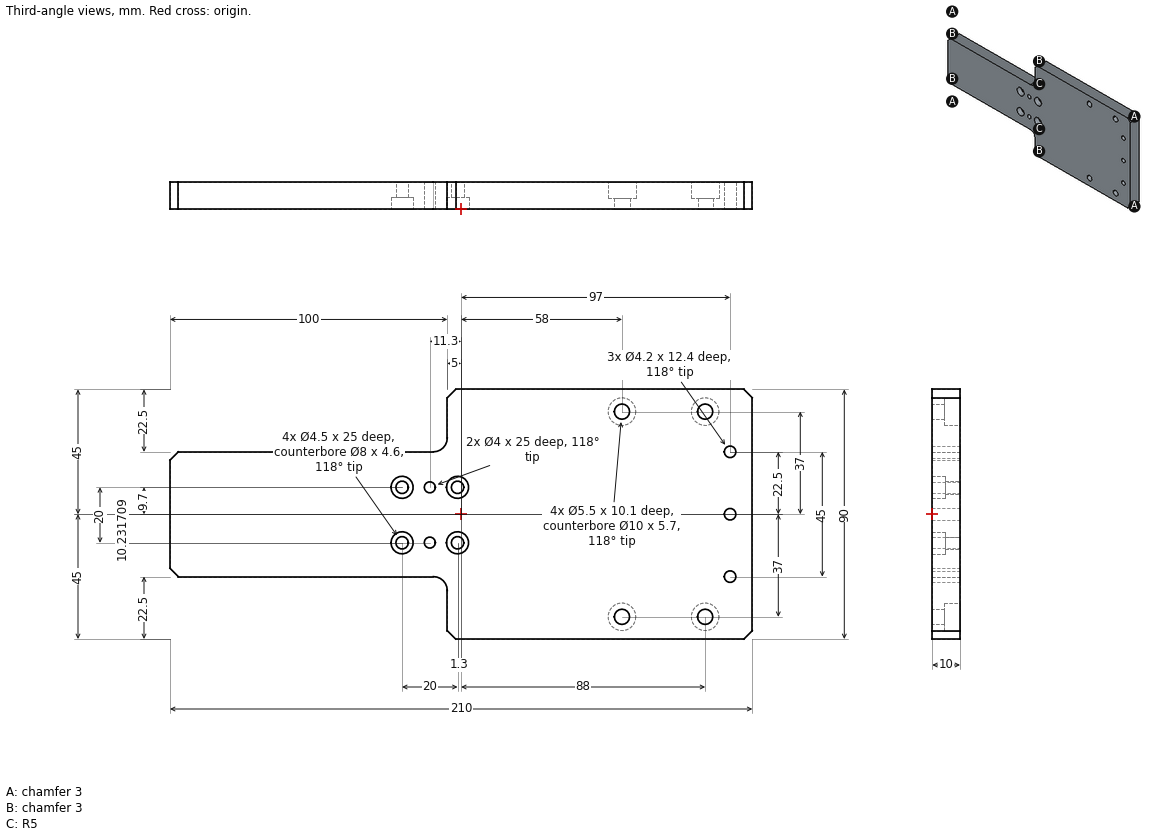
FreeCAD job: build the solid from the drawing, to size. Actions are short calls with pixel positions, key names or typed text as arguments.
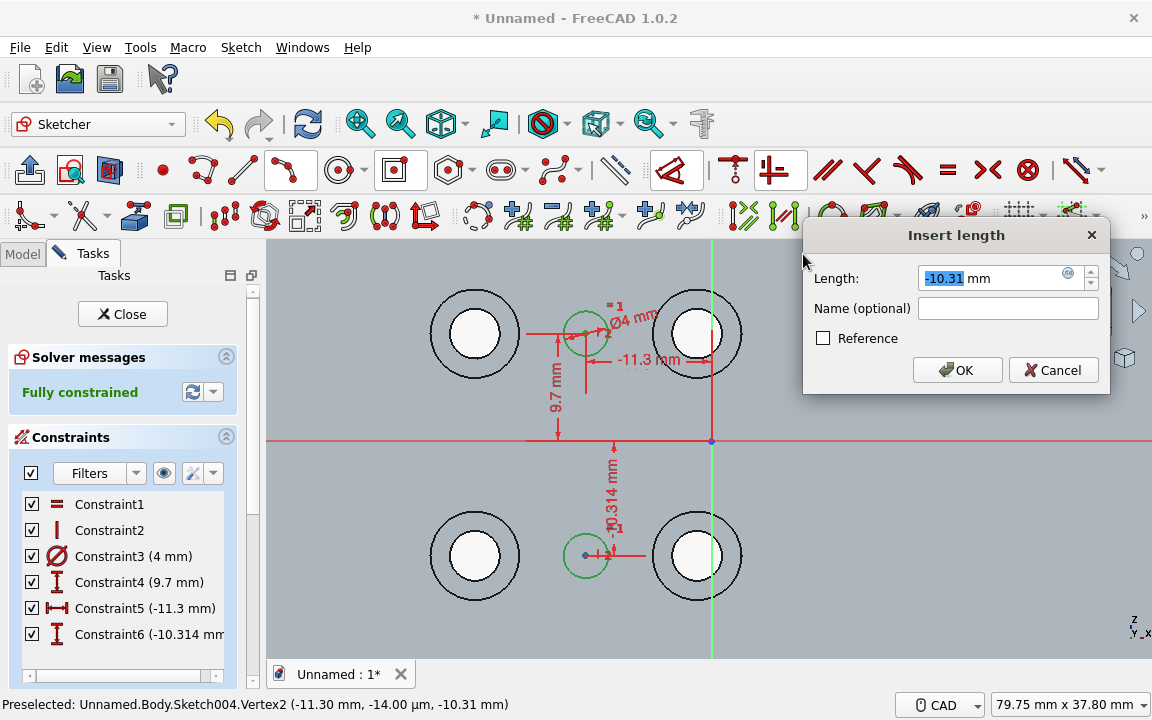
text(-10.231709)
key(Return)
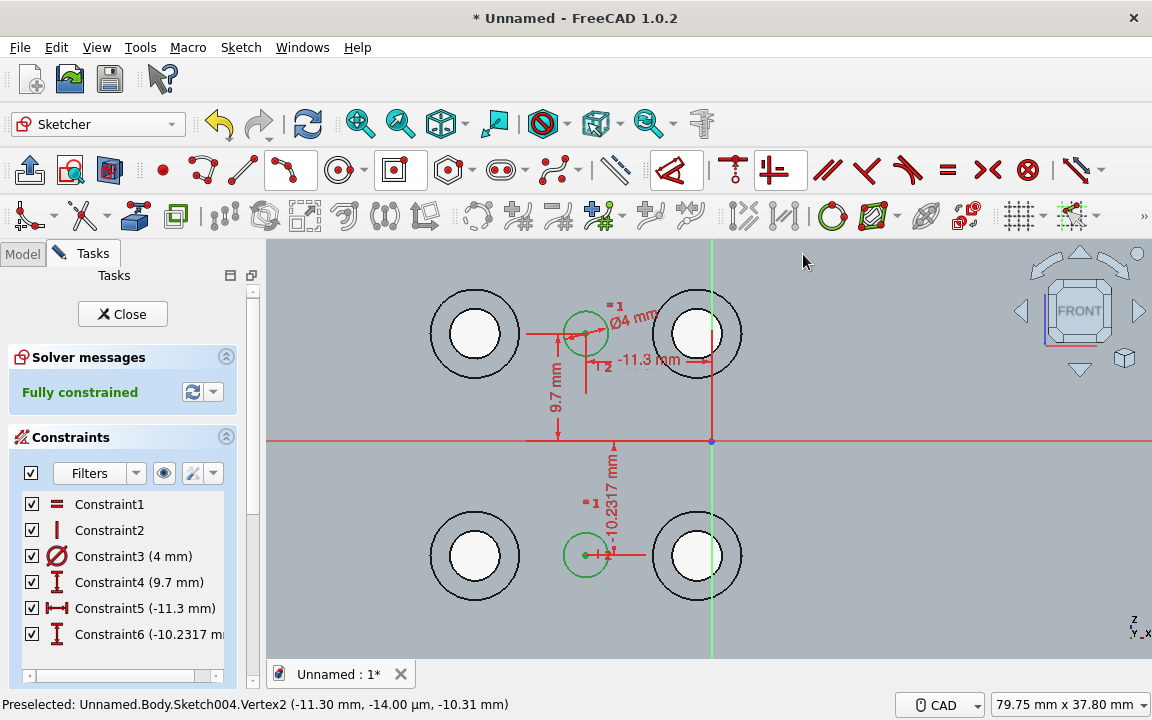
click(123, 314)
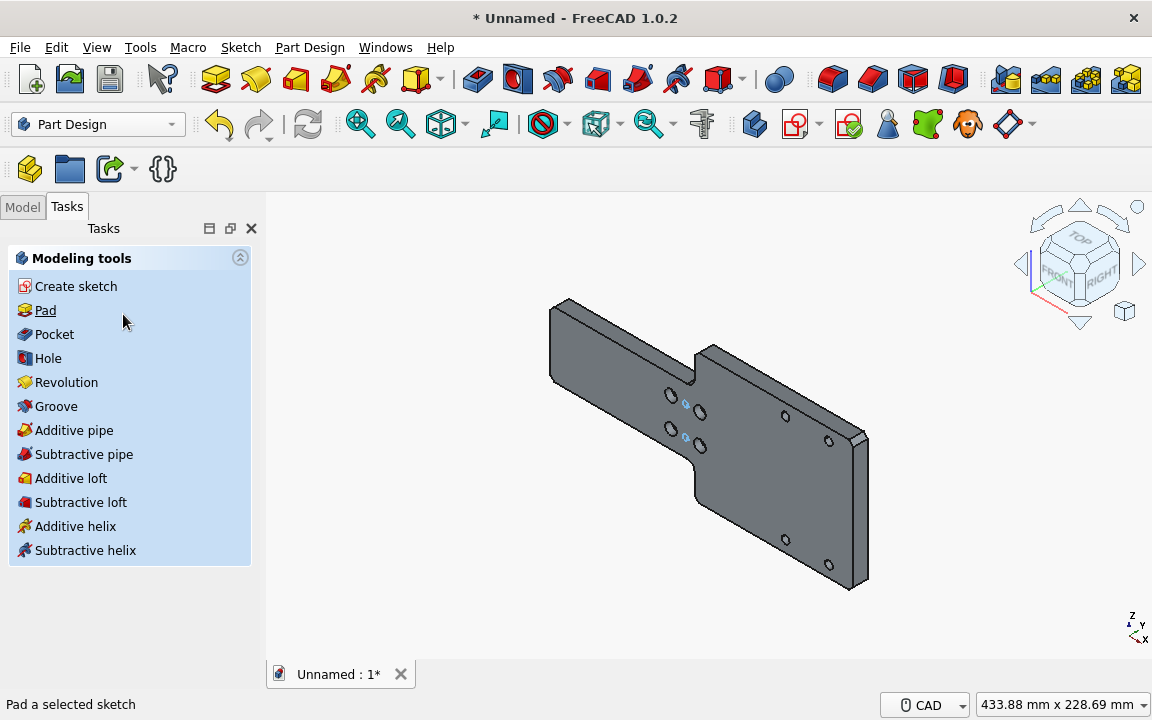
click(518, 80)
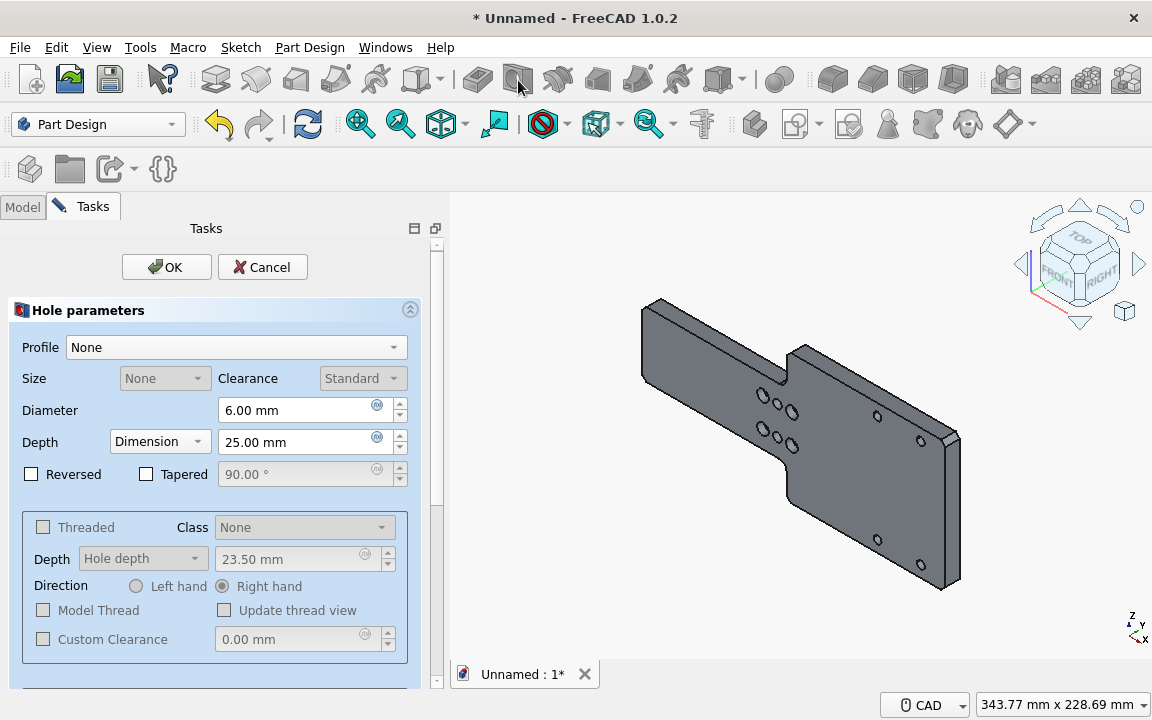
triple_click(305, 410)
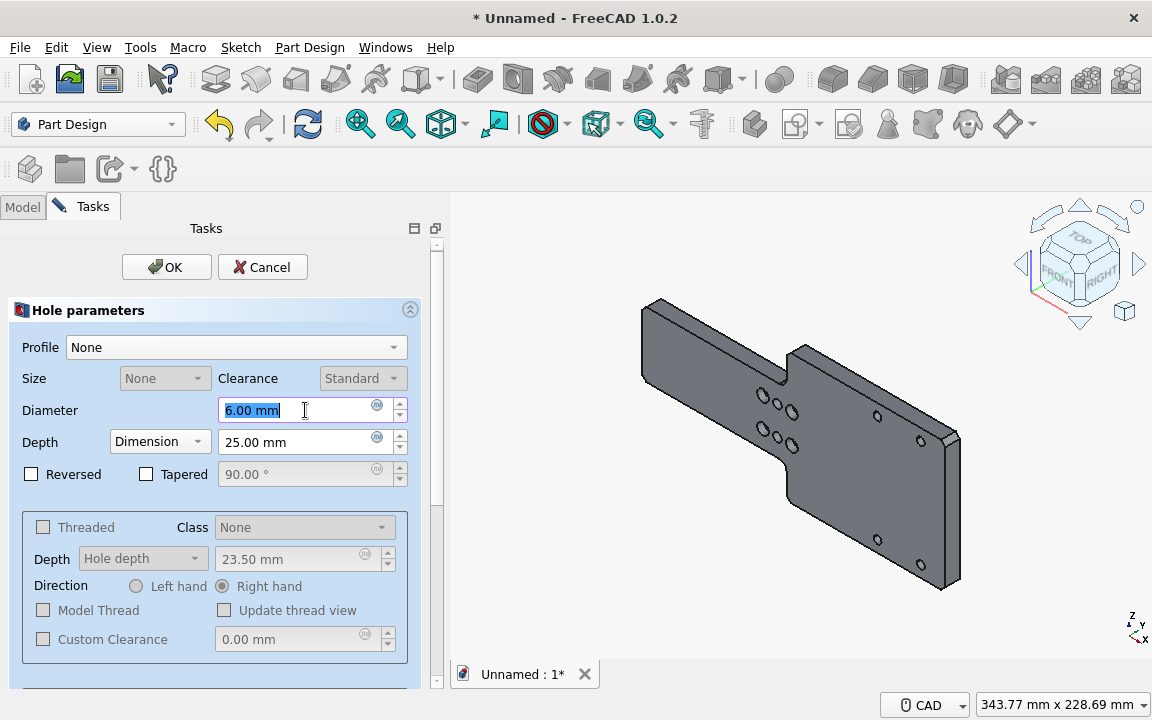
text(4)
key(Tab)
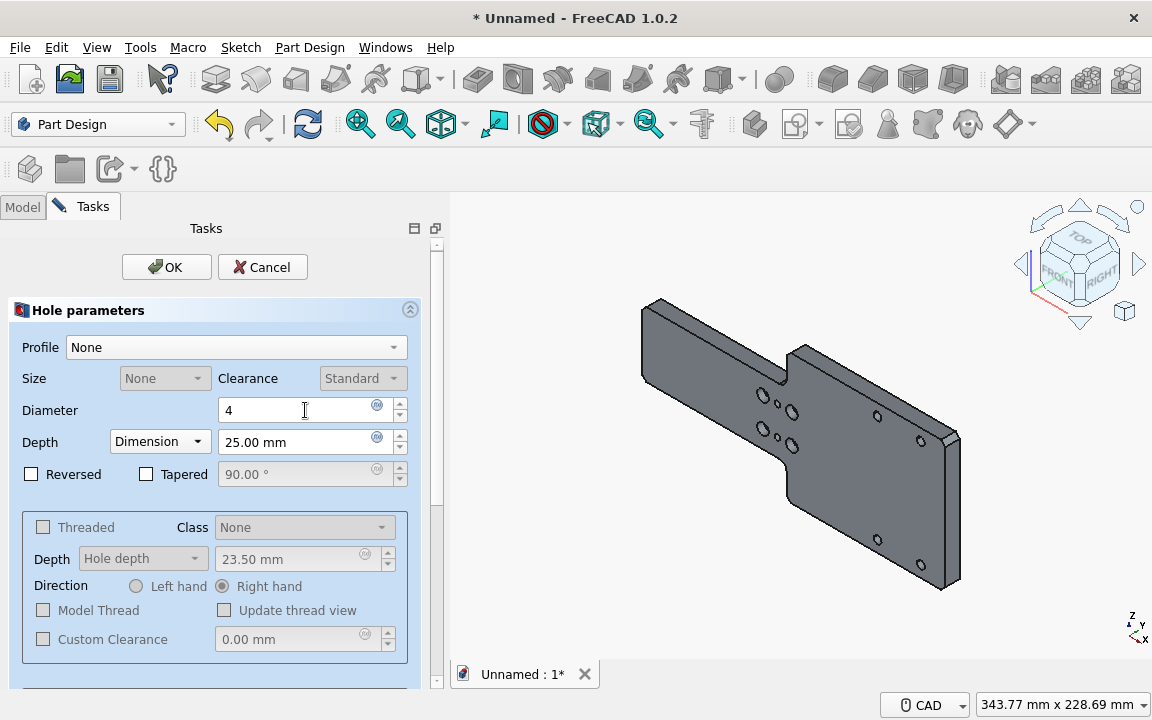
triple_click(305, 442)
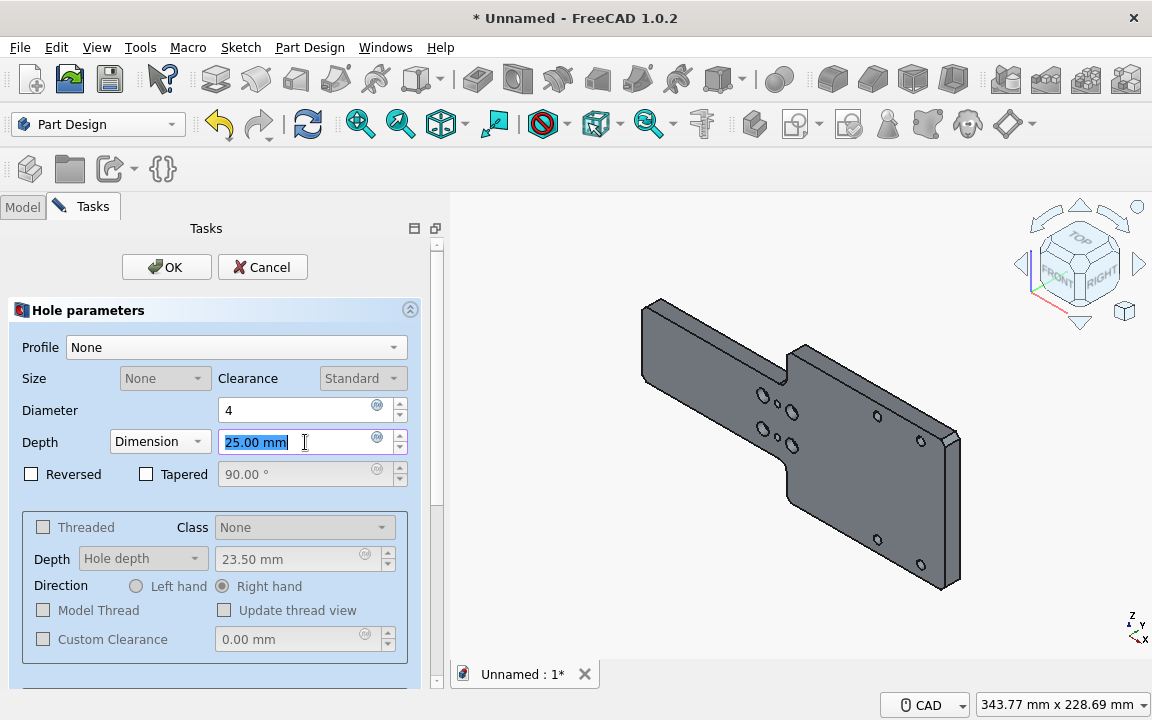
text(25)
key(Tab)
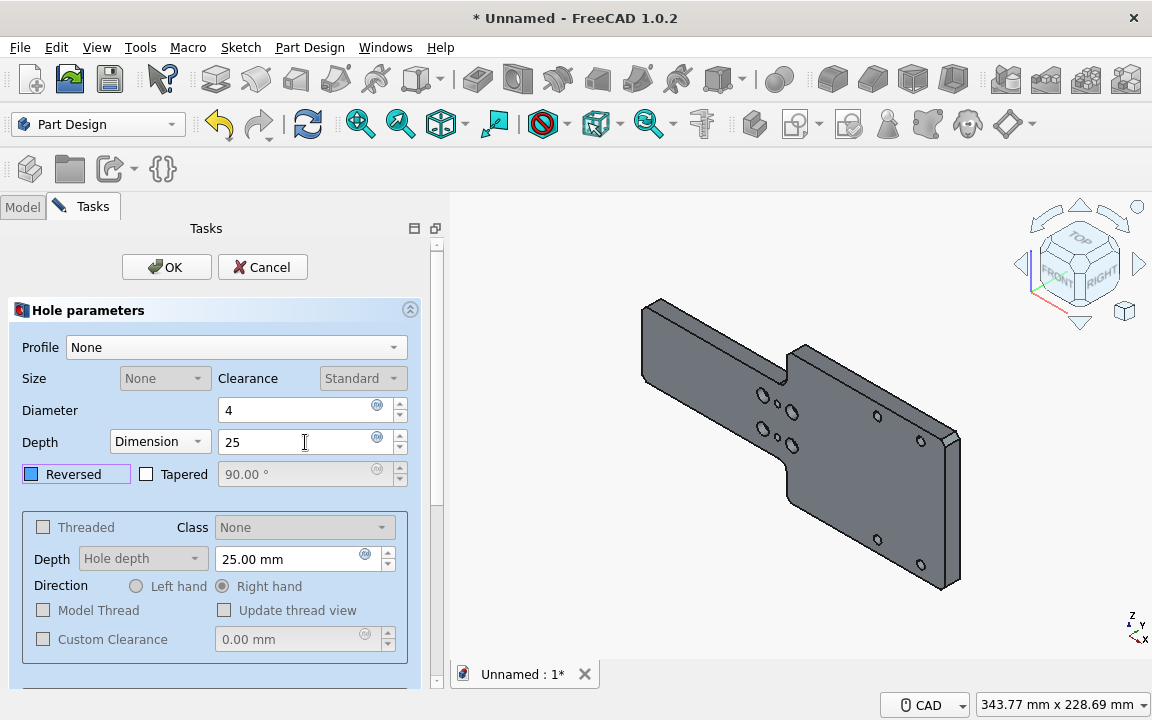
click(167, 267)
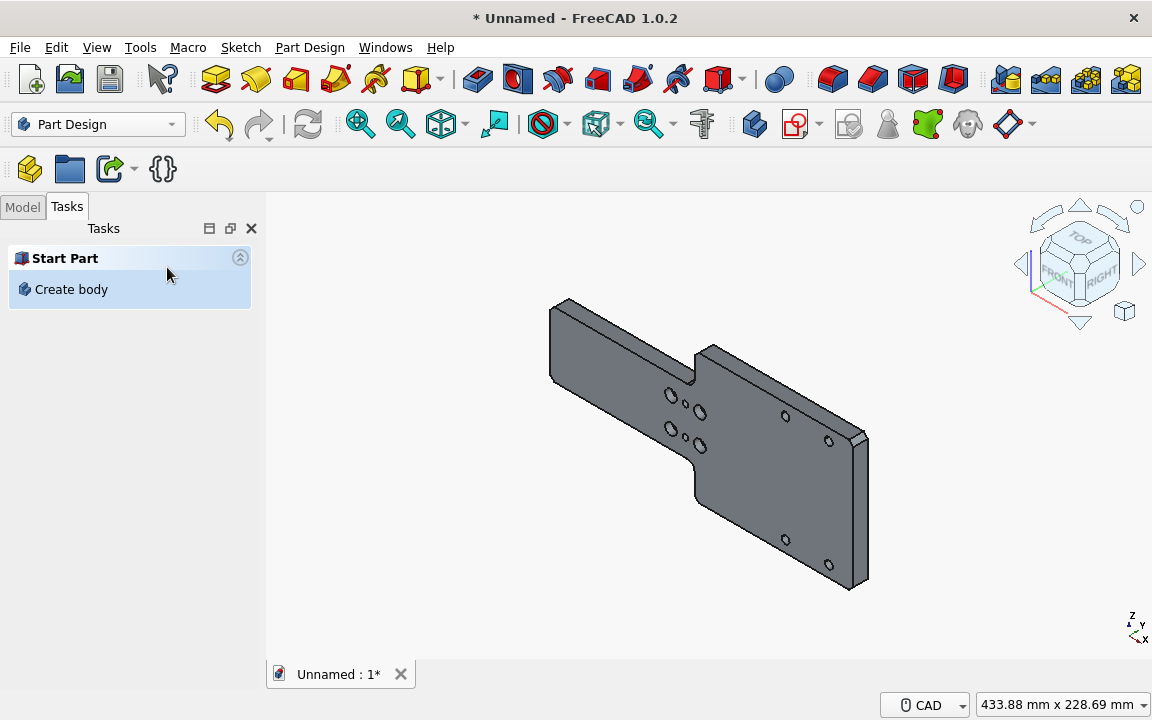
key(4)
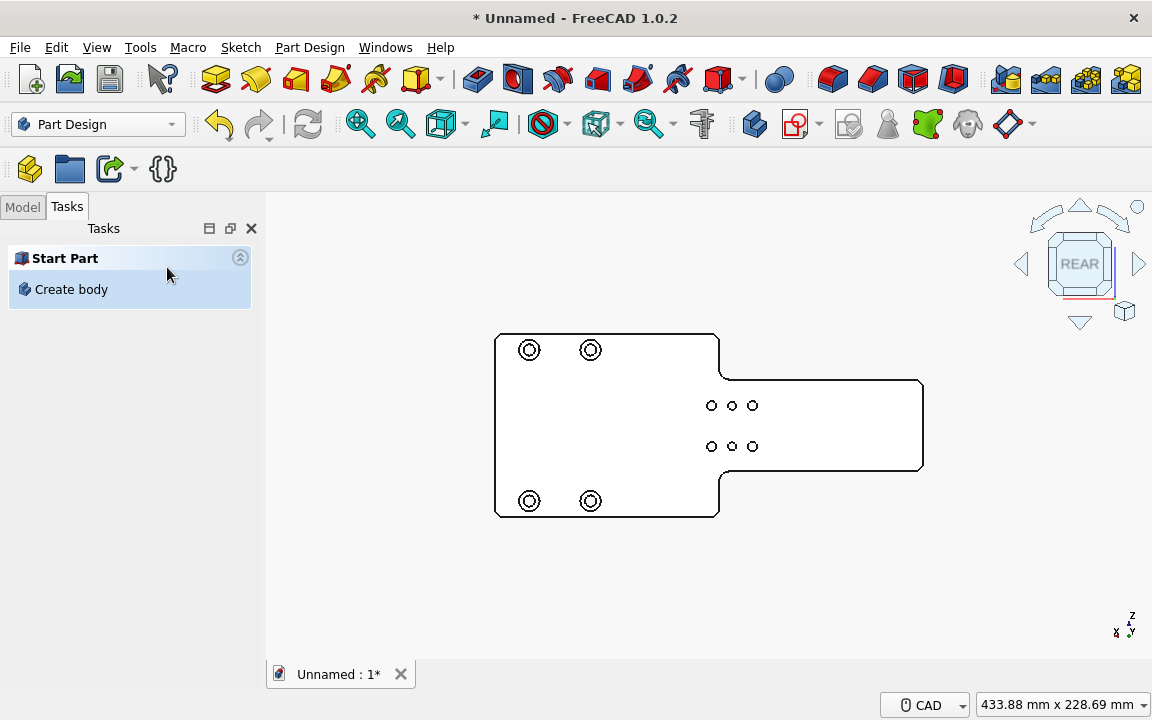
click(586, 424)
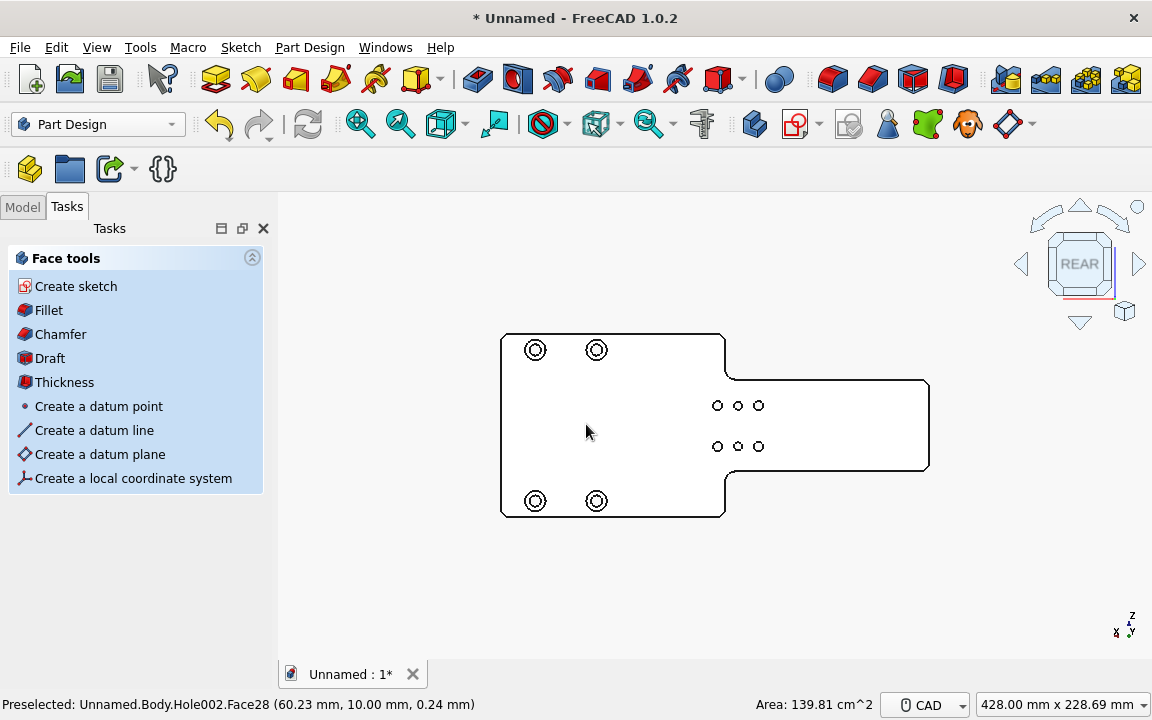
click(796, 124)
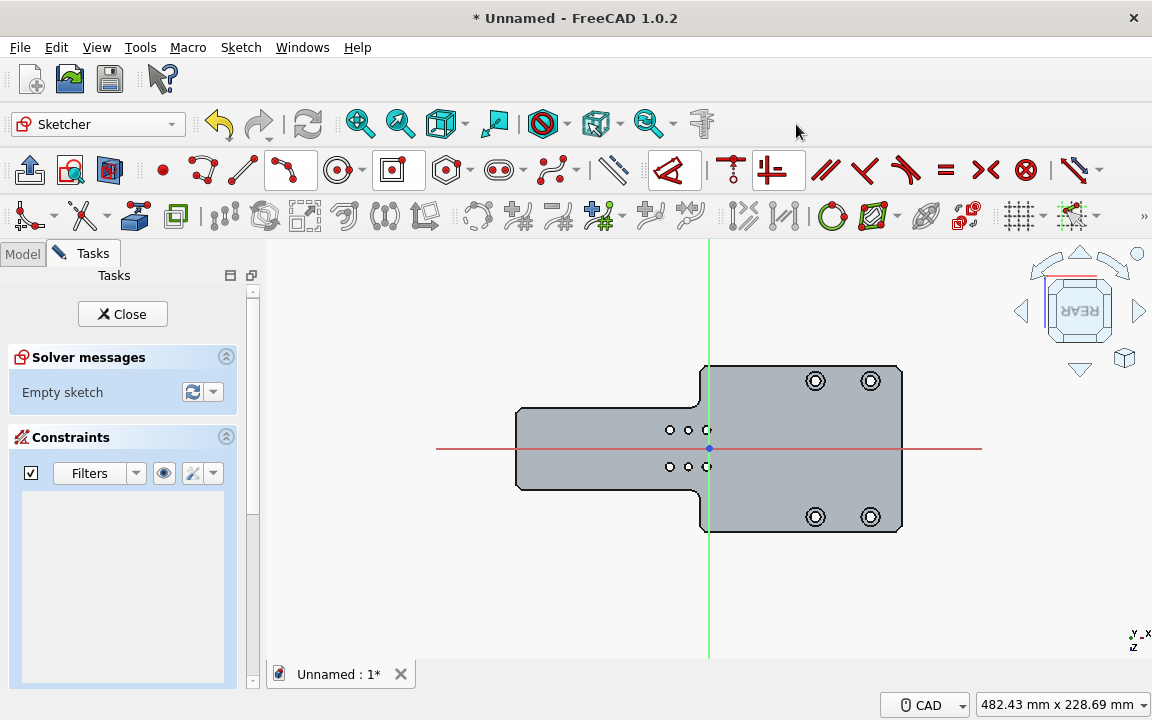
scroll(893, 449, up, 5)